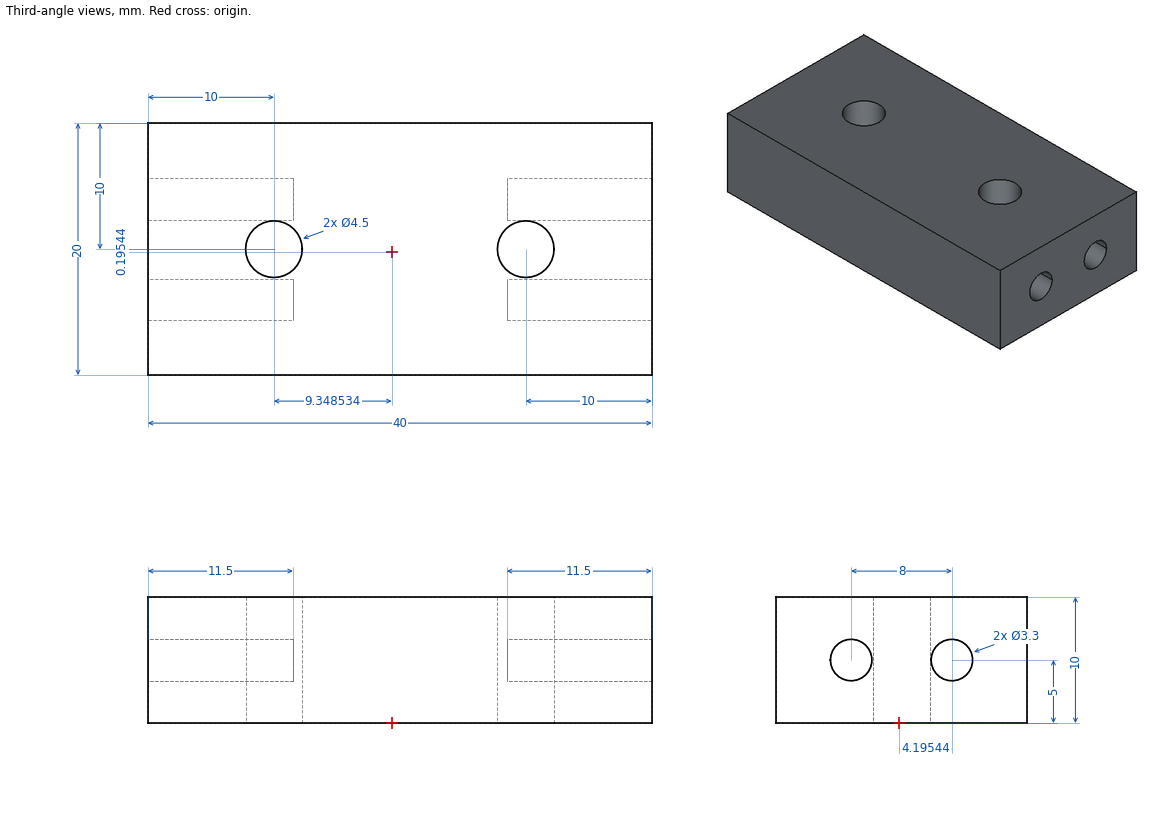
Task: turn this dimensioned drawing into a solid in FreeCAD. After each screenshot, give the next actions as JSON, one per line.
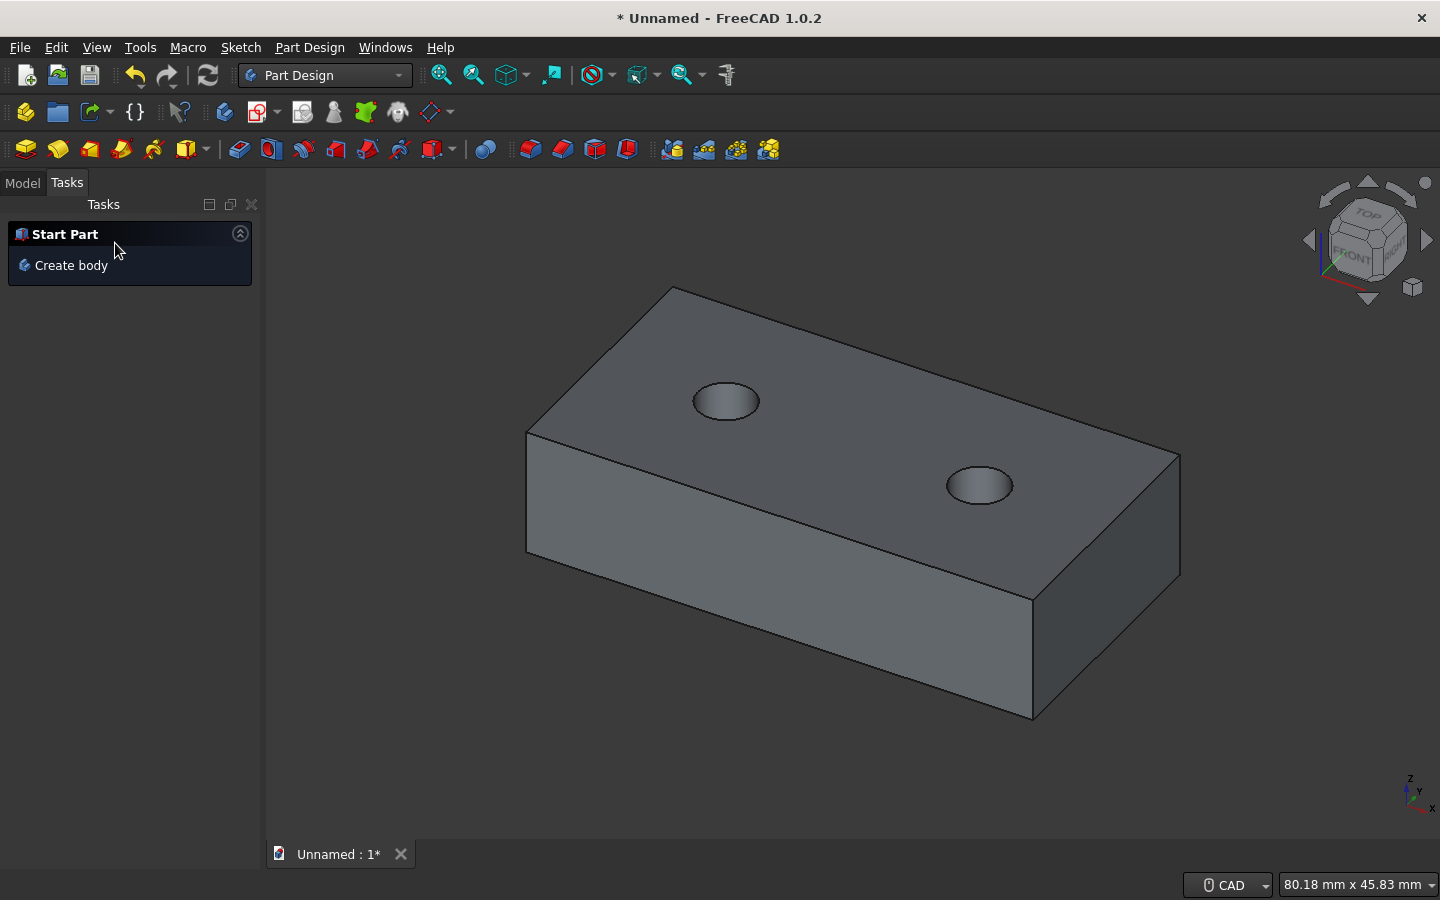
{"action": "key", "text": "6"}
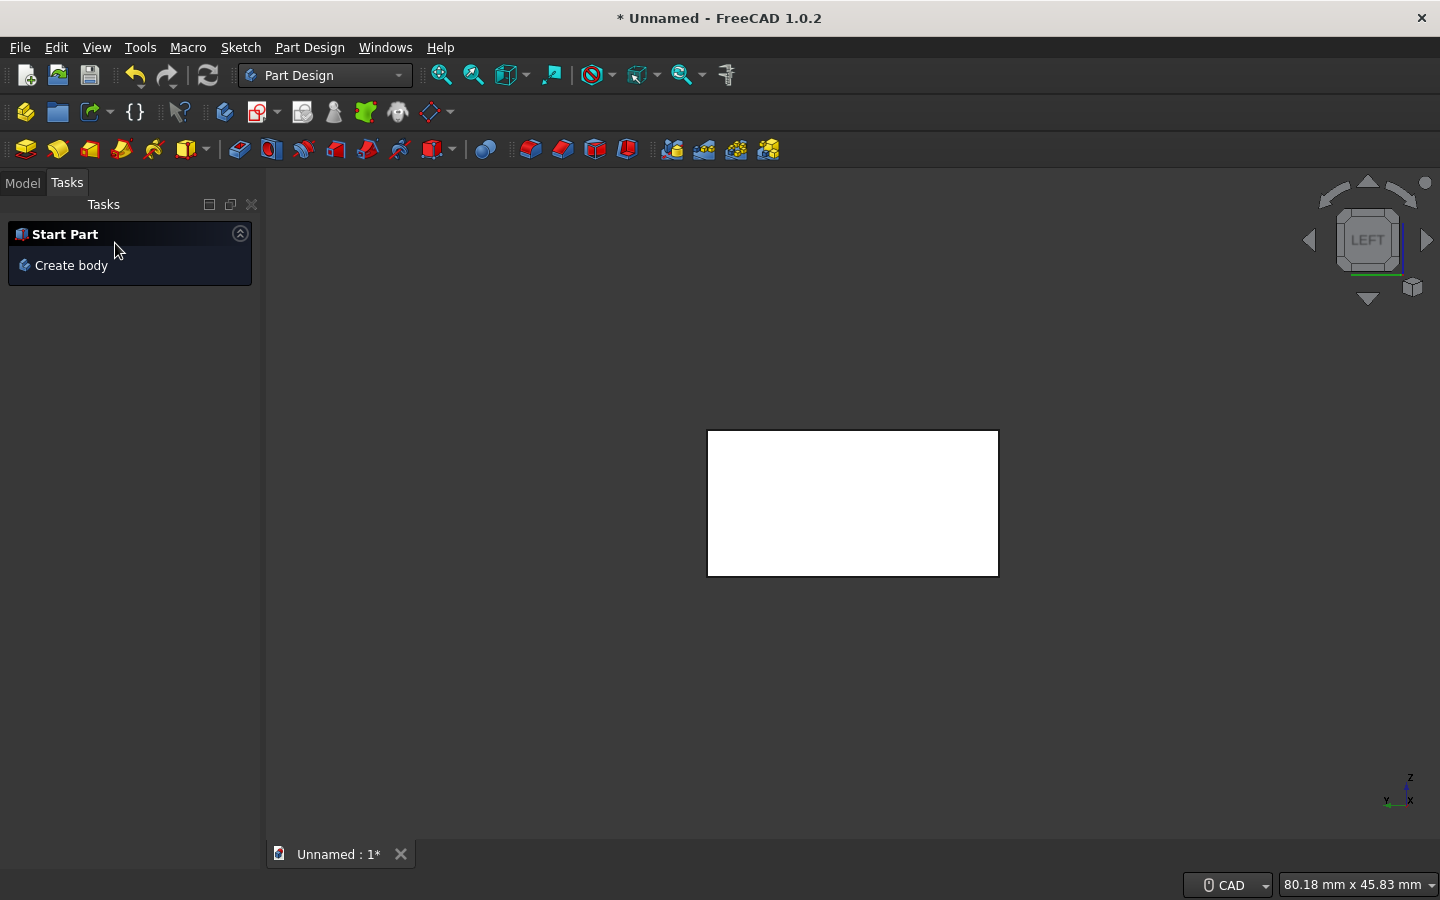
{"action": "key", "text": "v f"}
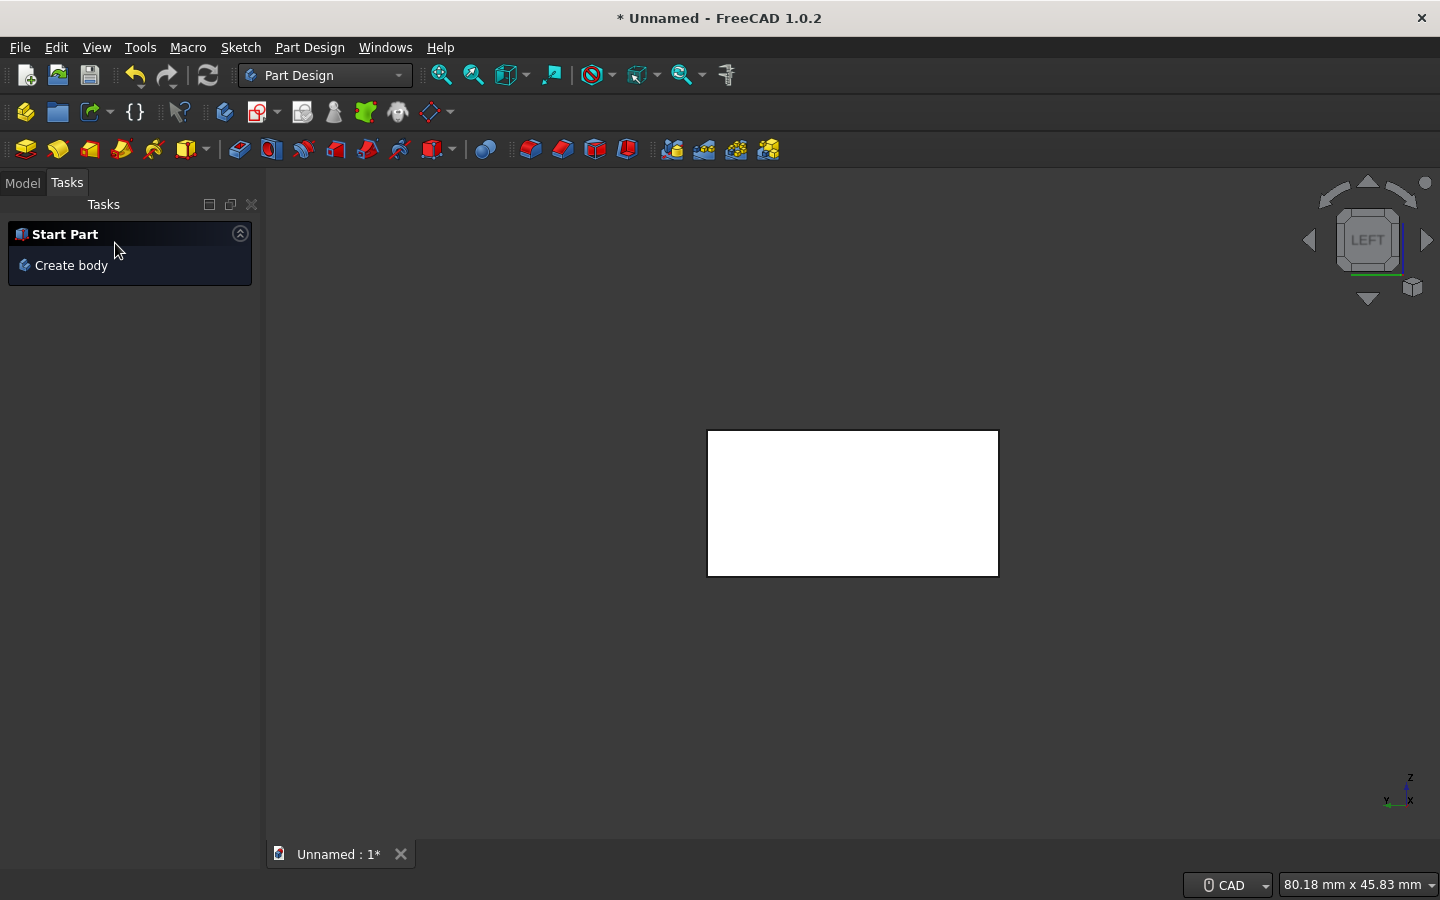
{"action": "left_click", "coordinate": [811, 502]}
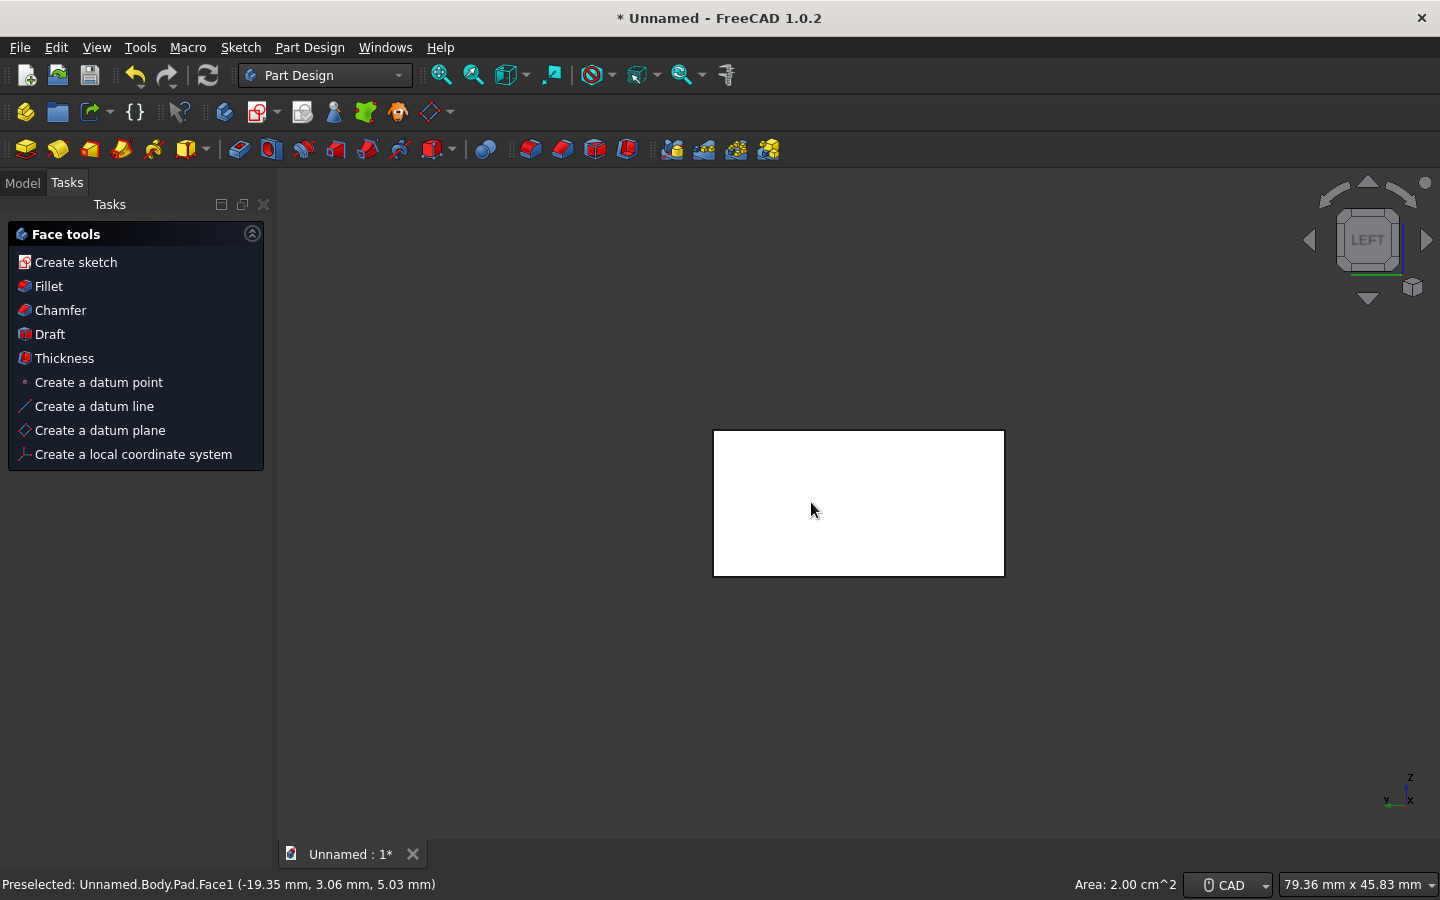
{"action": "left_click", "coordinate": [258, 112]}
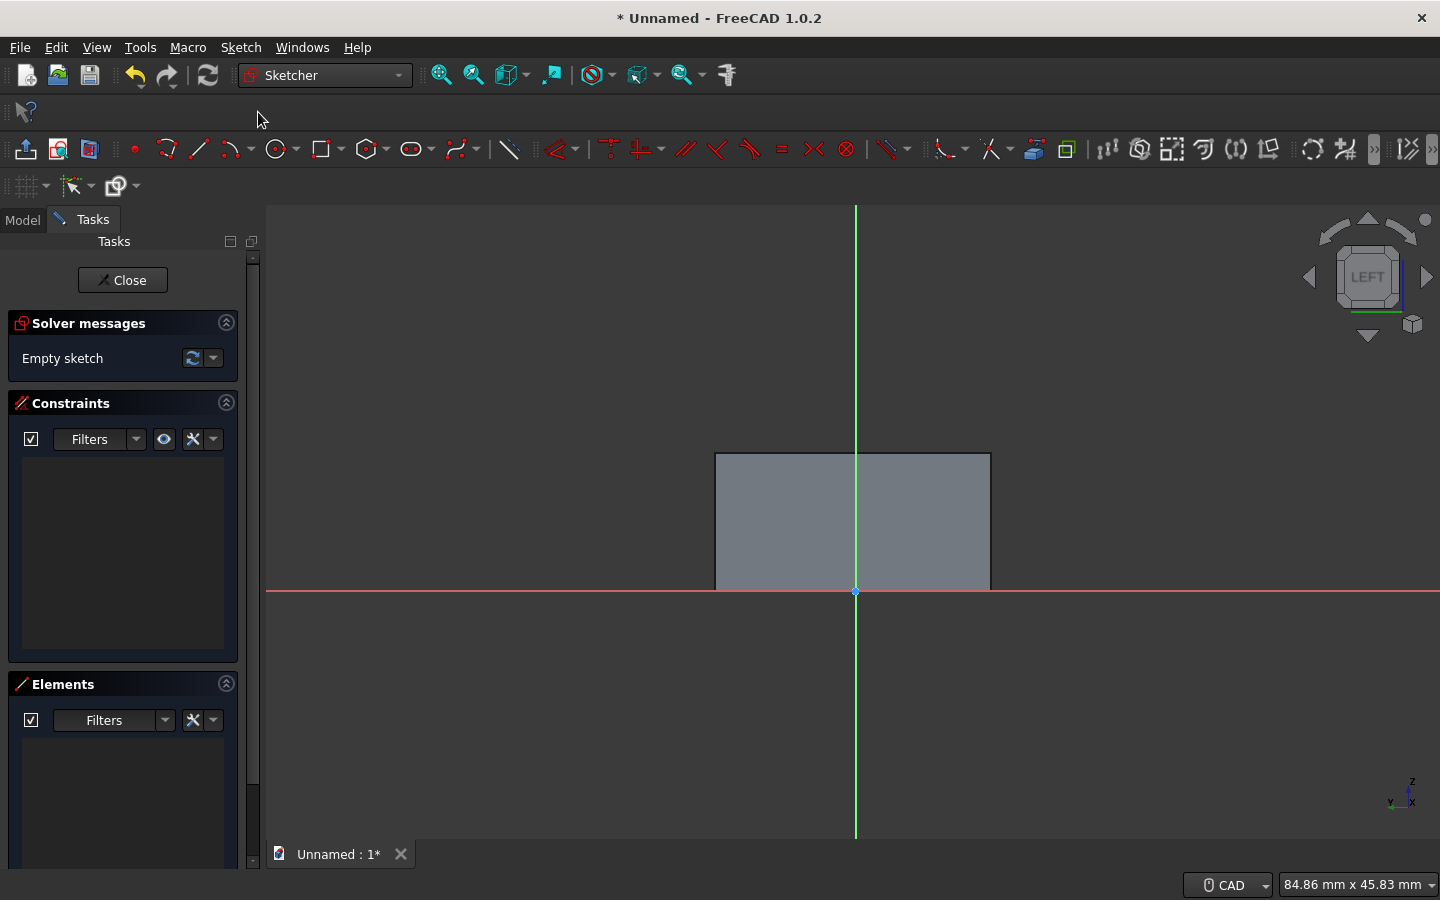
{"action": "scroll", "coordinate": [875, 553], "scroll_direction": "up", "scroll_amount": 7}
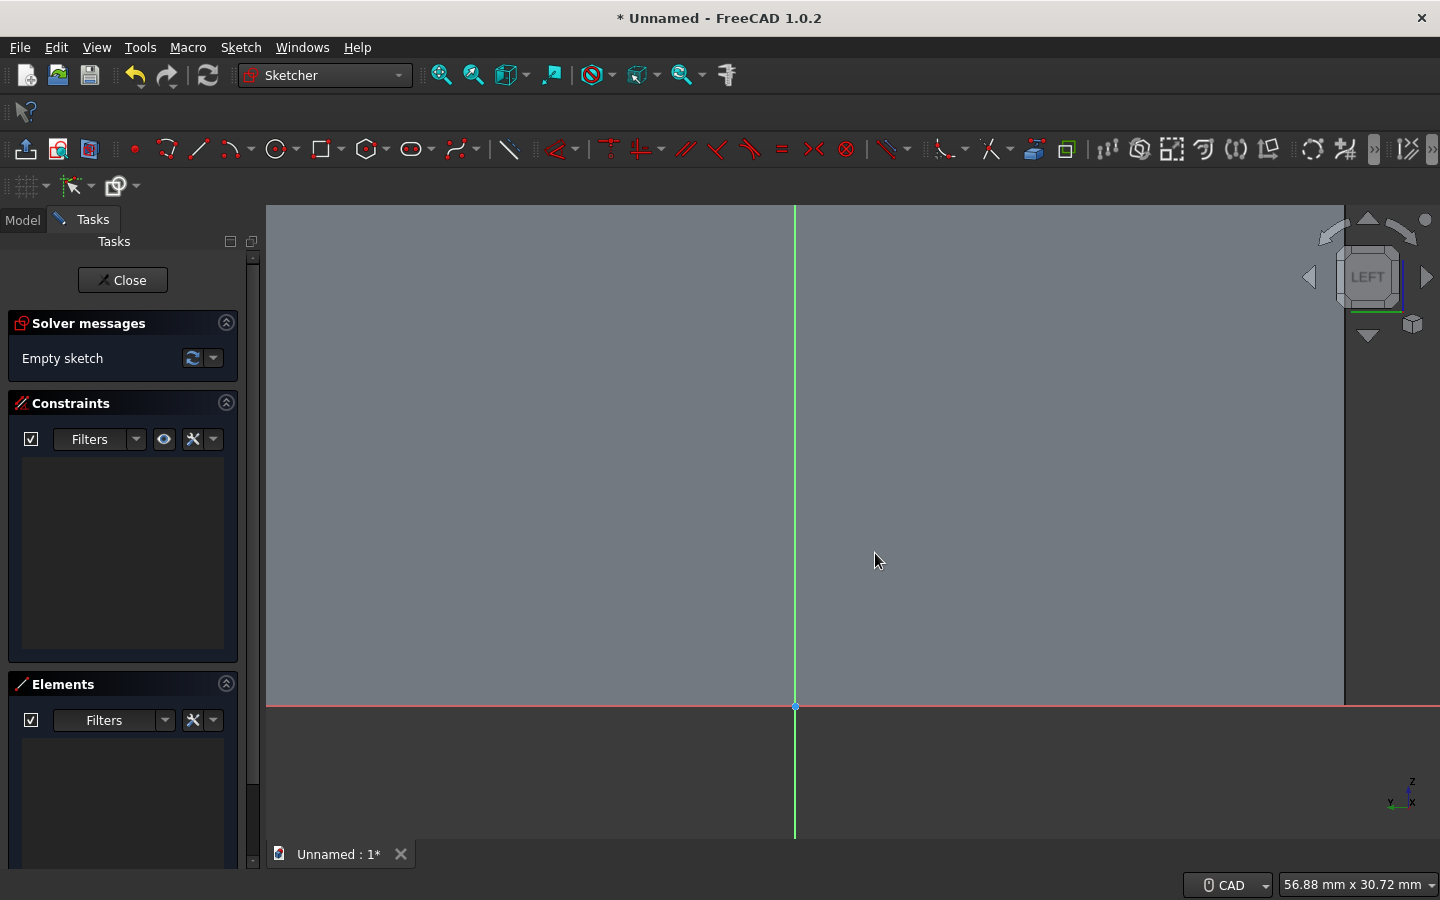
{"action": "key", "text": "g c"}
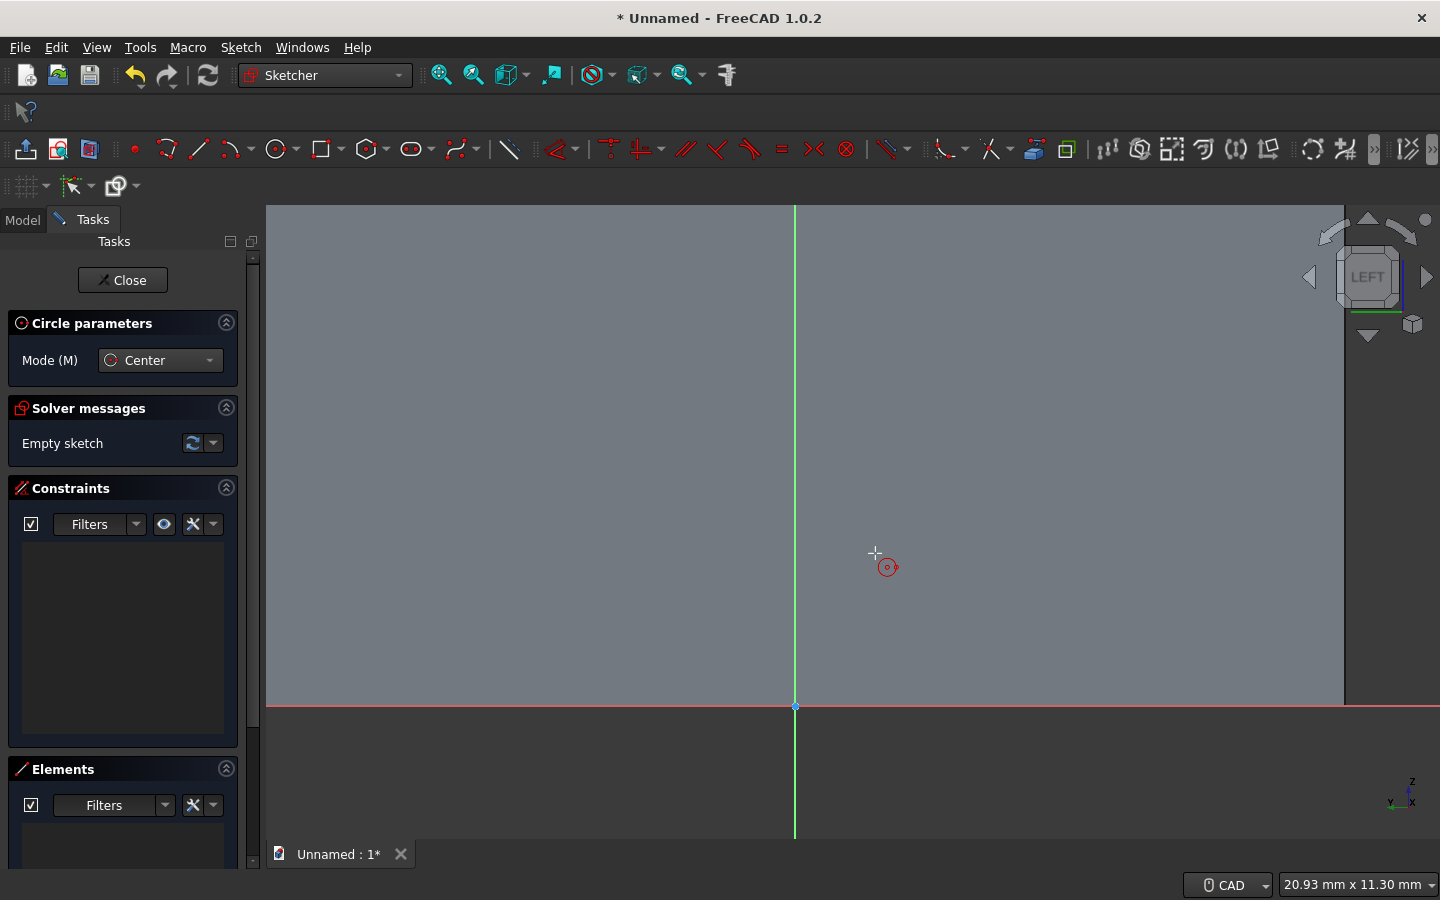
{"action": "left_click", "coordinate": [560, 426]}
{"action": "left_click", "coordinate": [625, 360]}